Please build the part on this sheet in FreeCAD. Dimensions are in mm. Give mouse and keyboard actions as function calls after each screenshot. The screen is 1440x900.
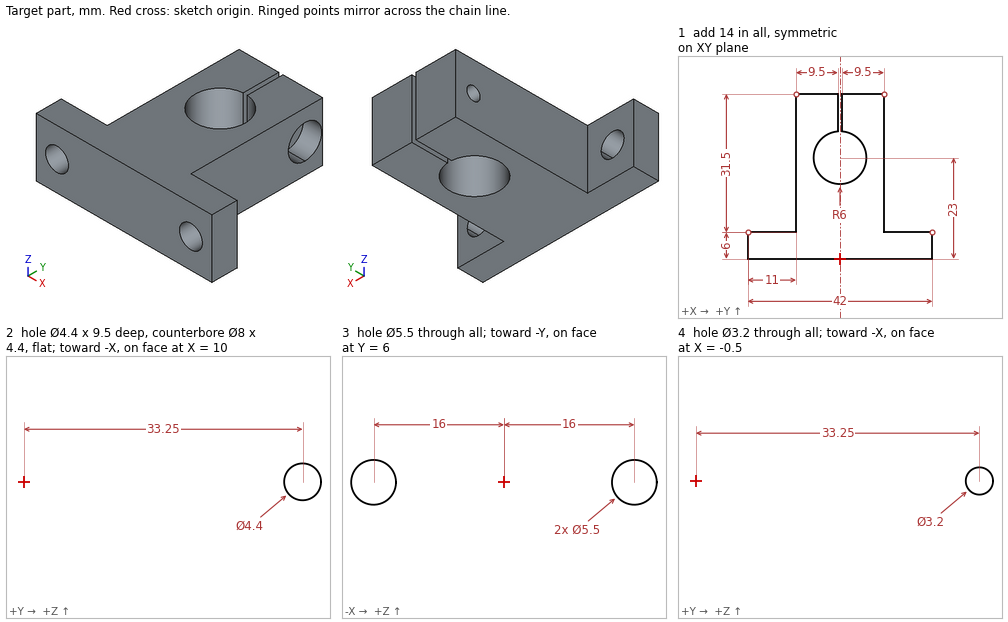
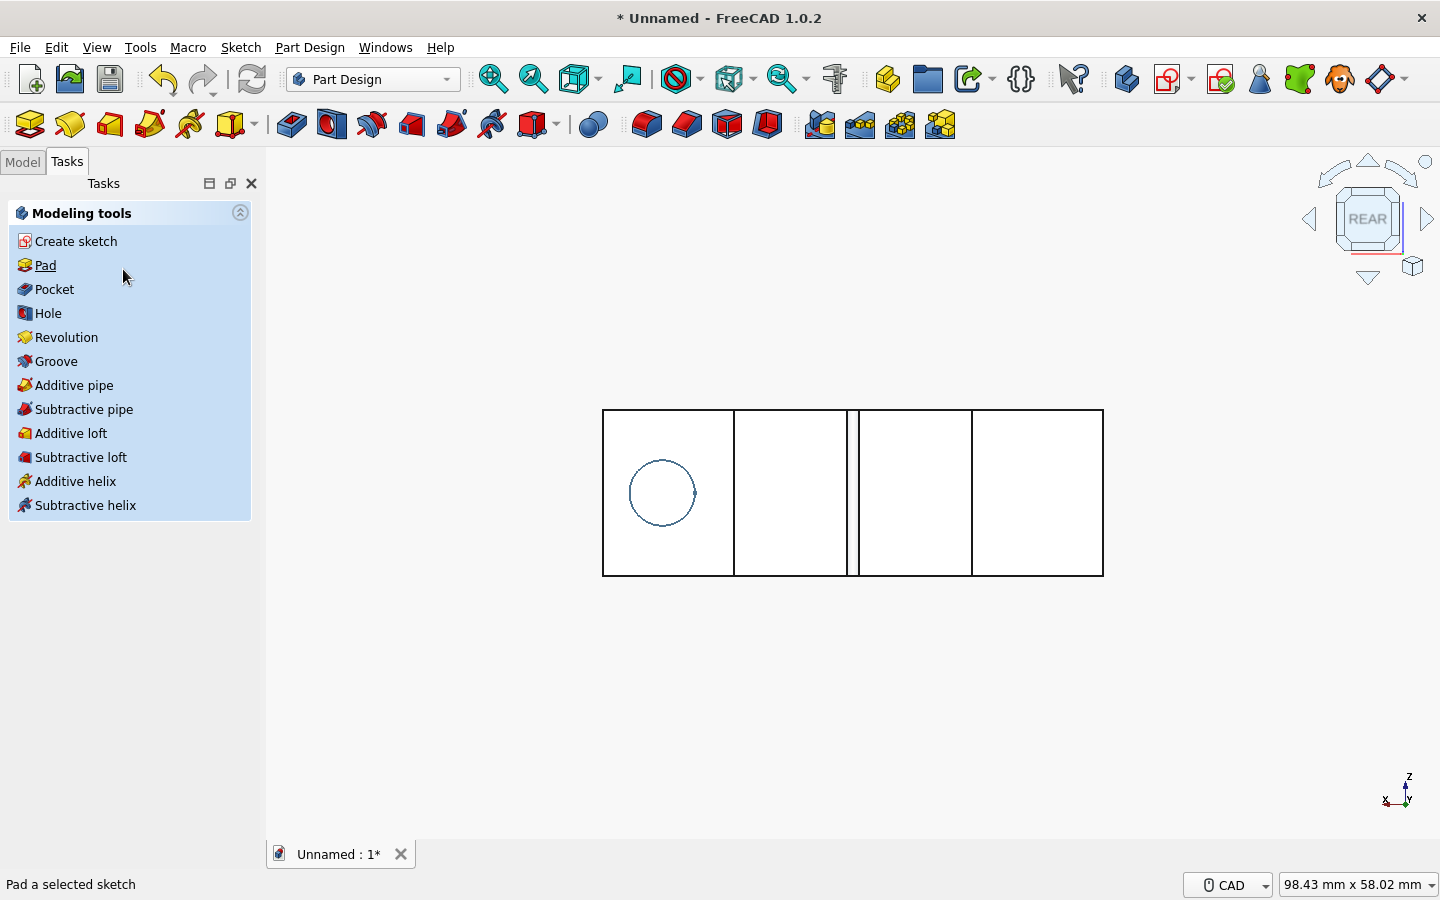
click(332, 124)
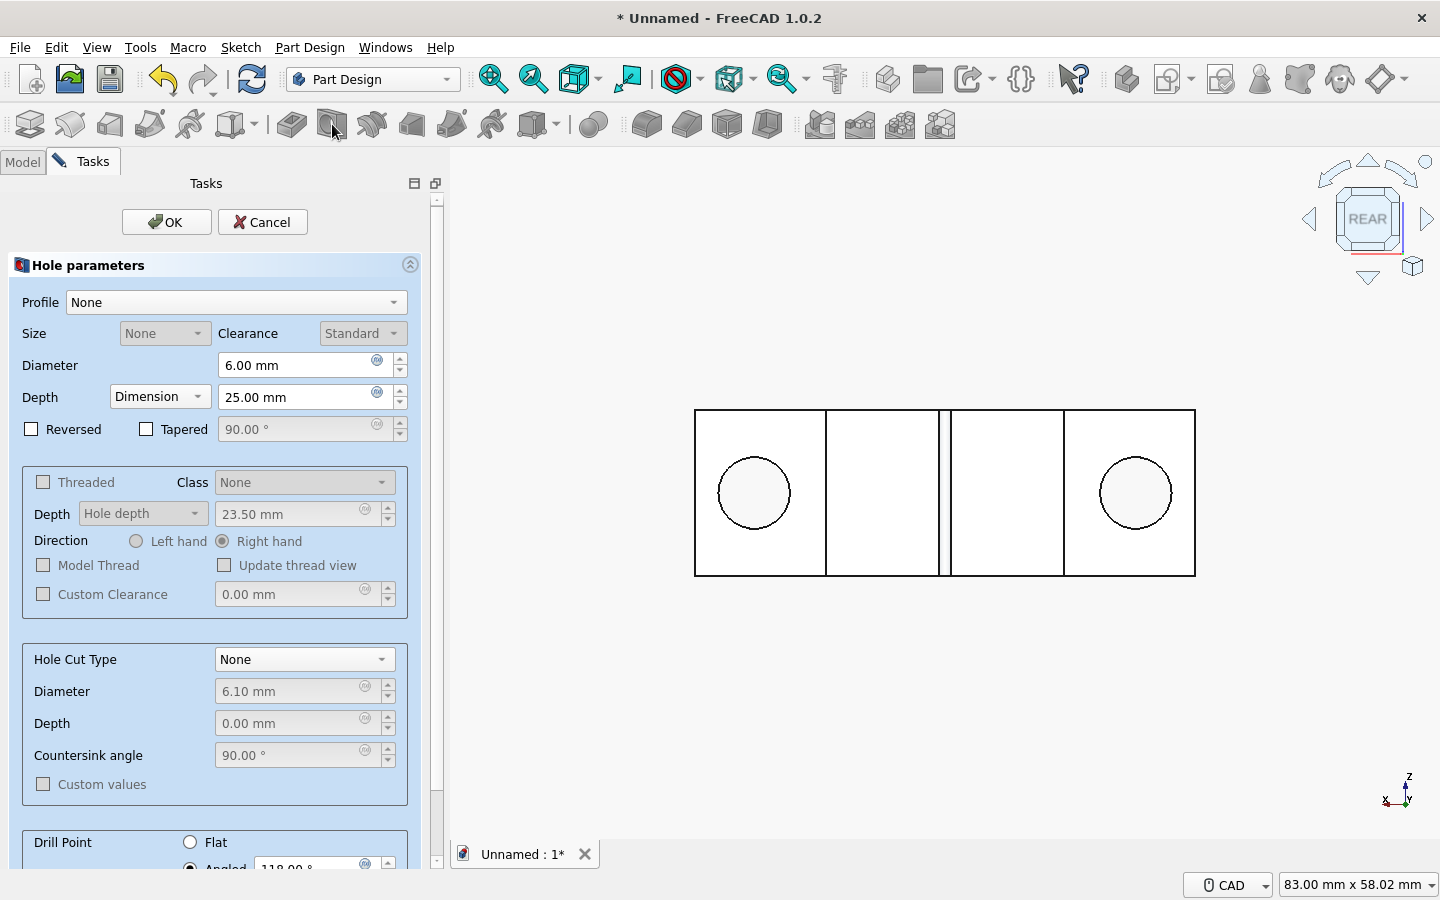
triple_click(305, 365)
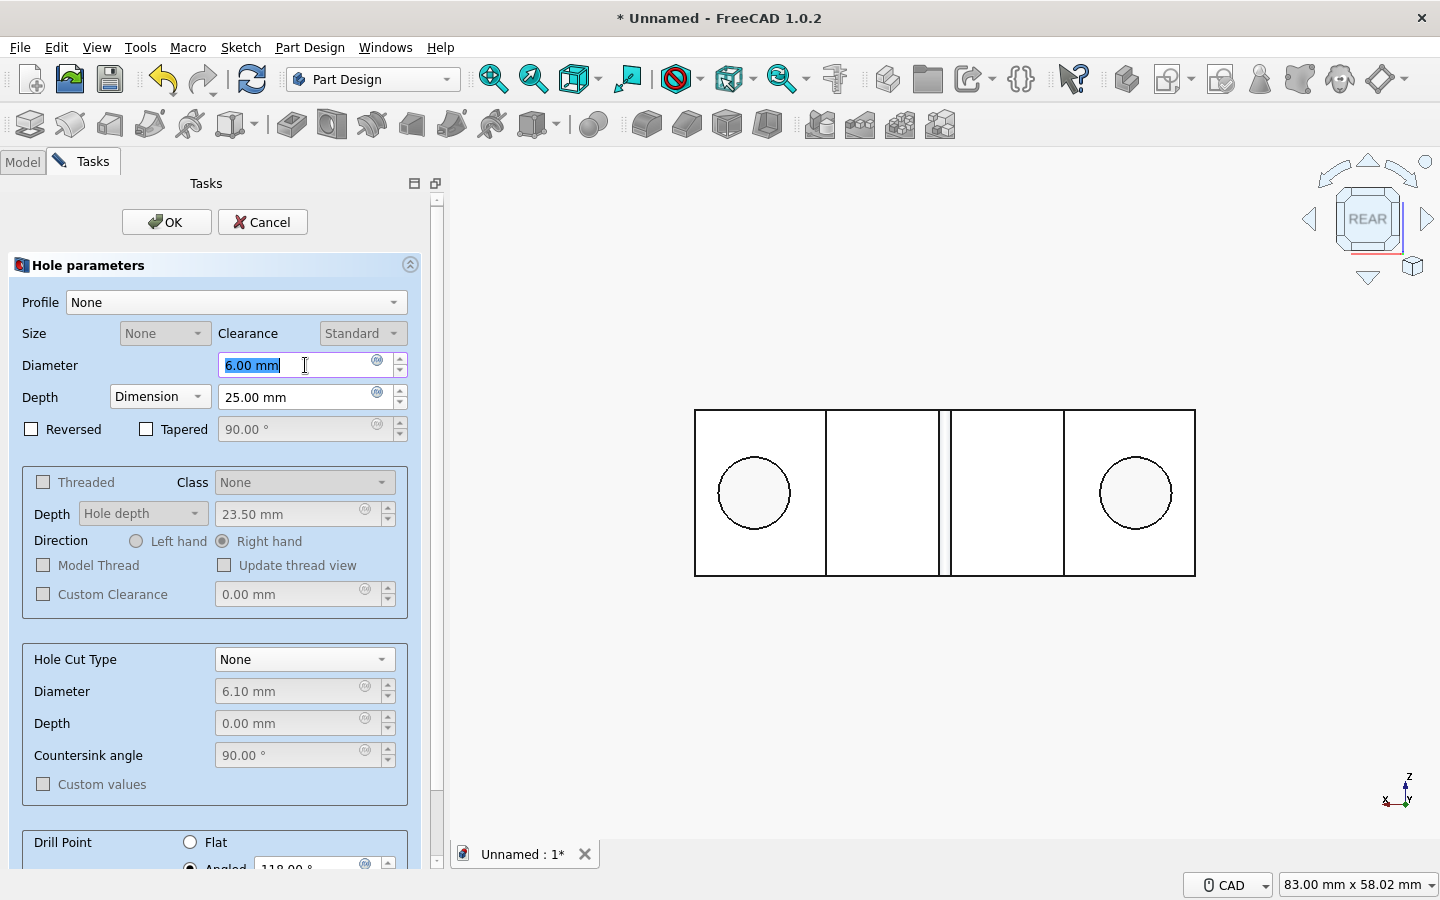
text(5.5)
key(Tab)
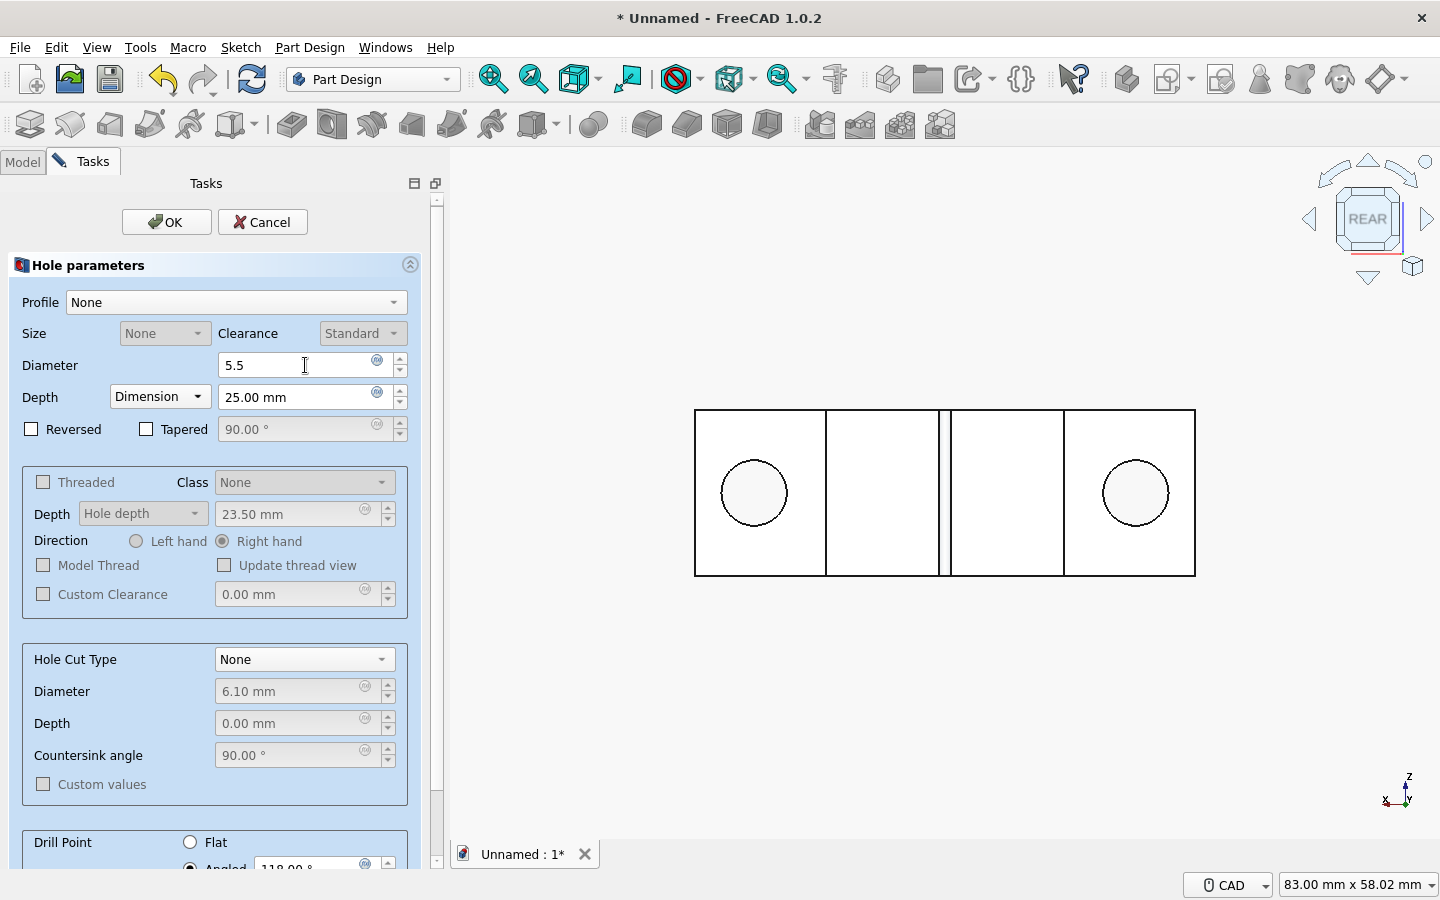
click(161, 396)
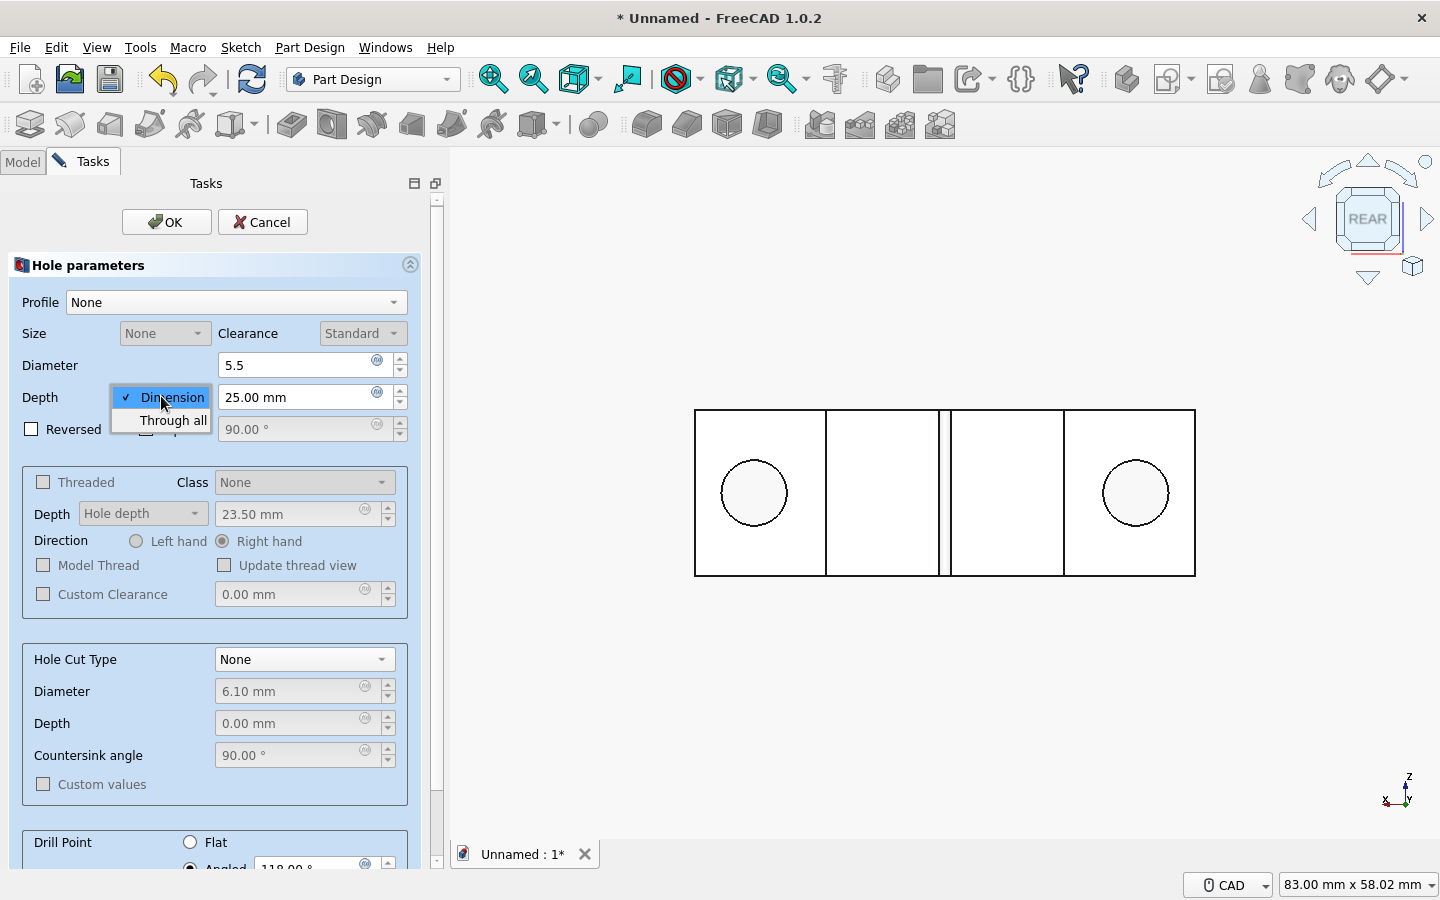
click(160, 420)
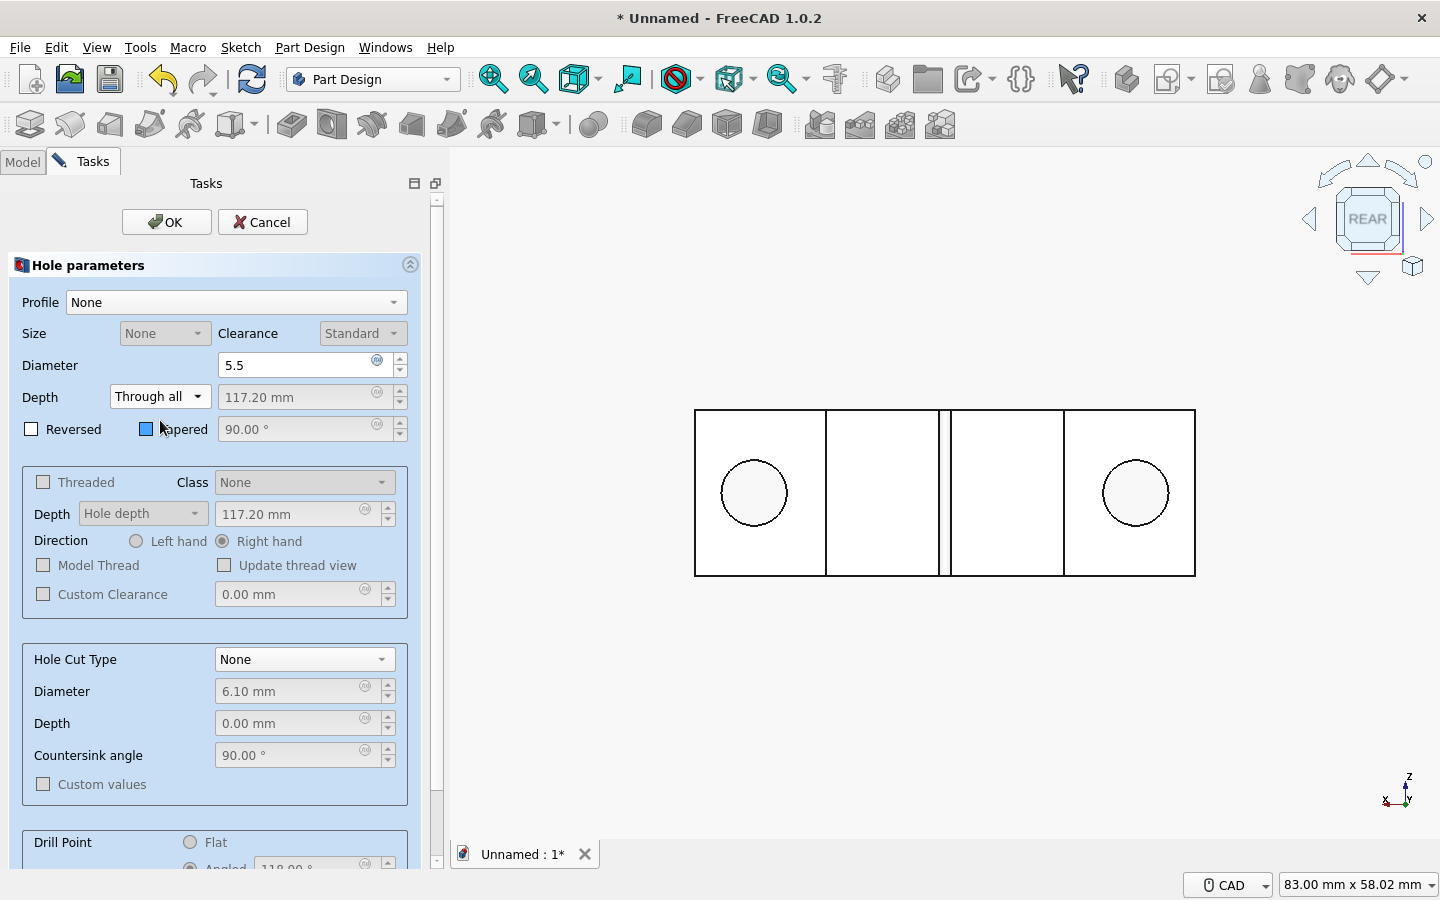
click(167, 222)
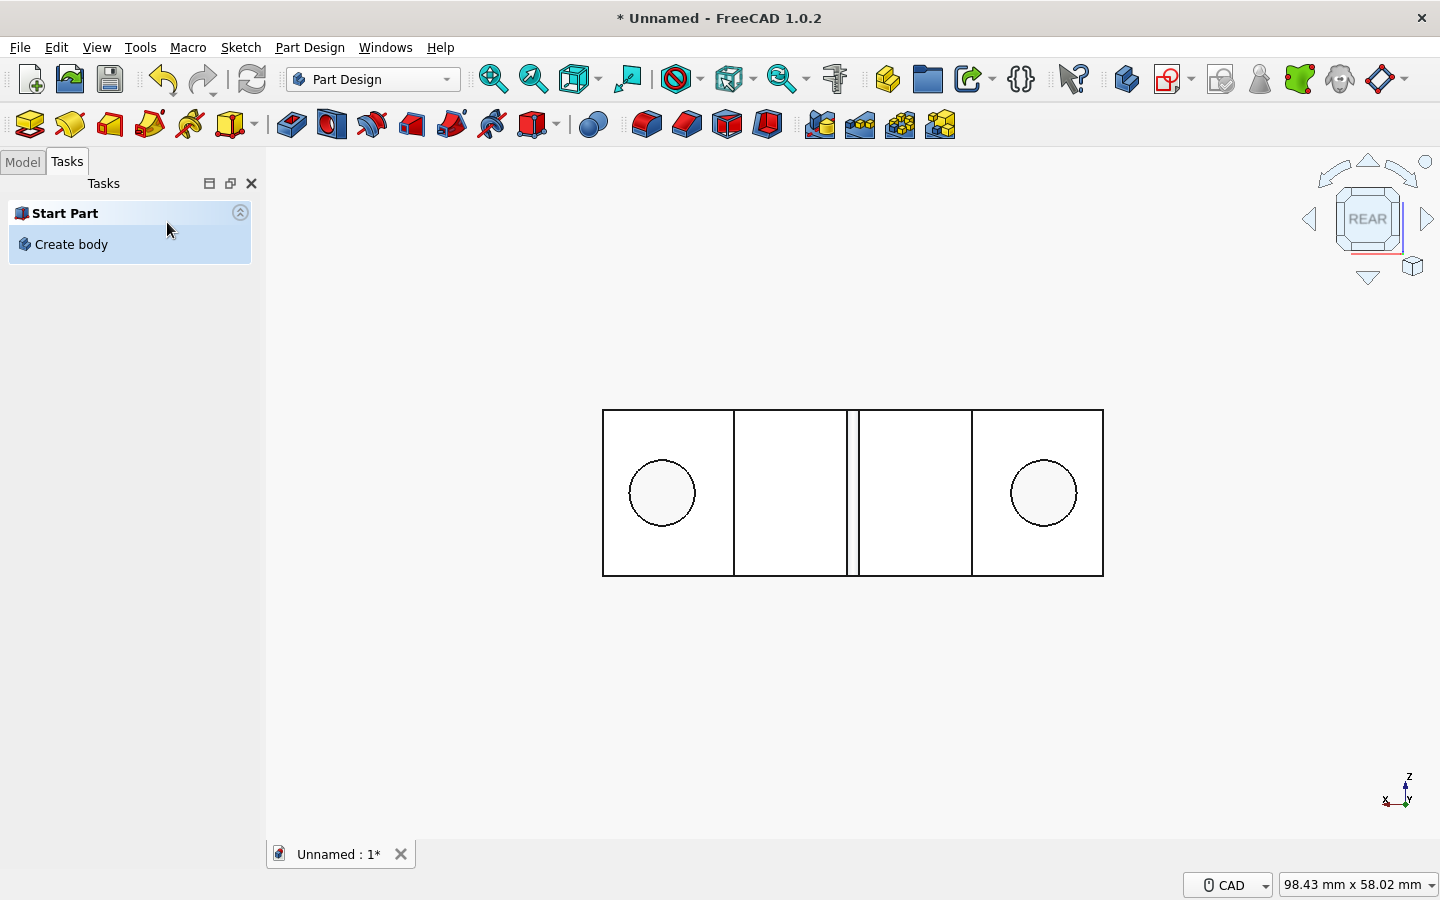
click(494, 80)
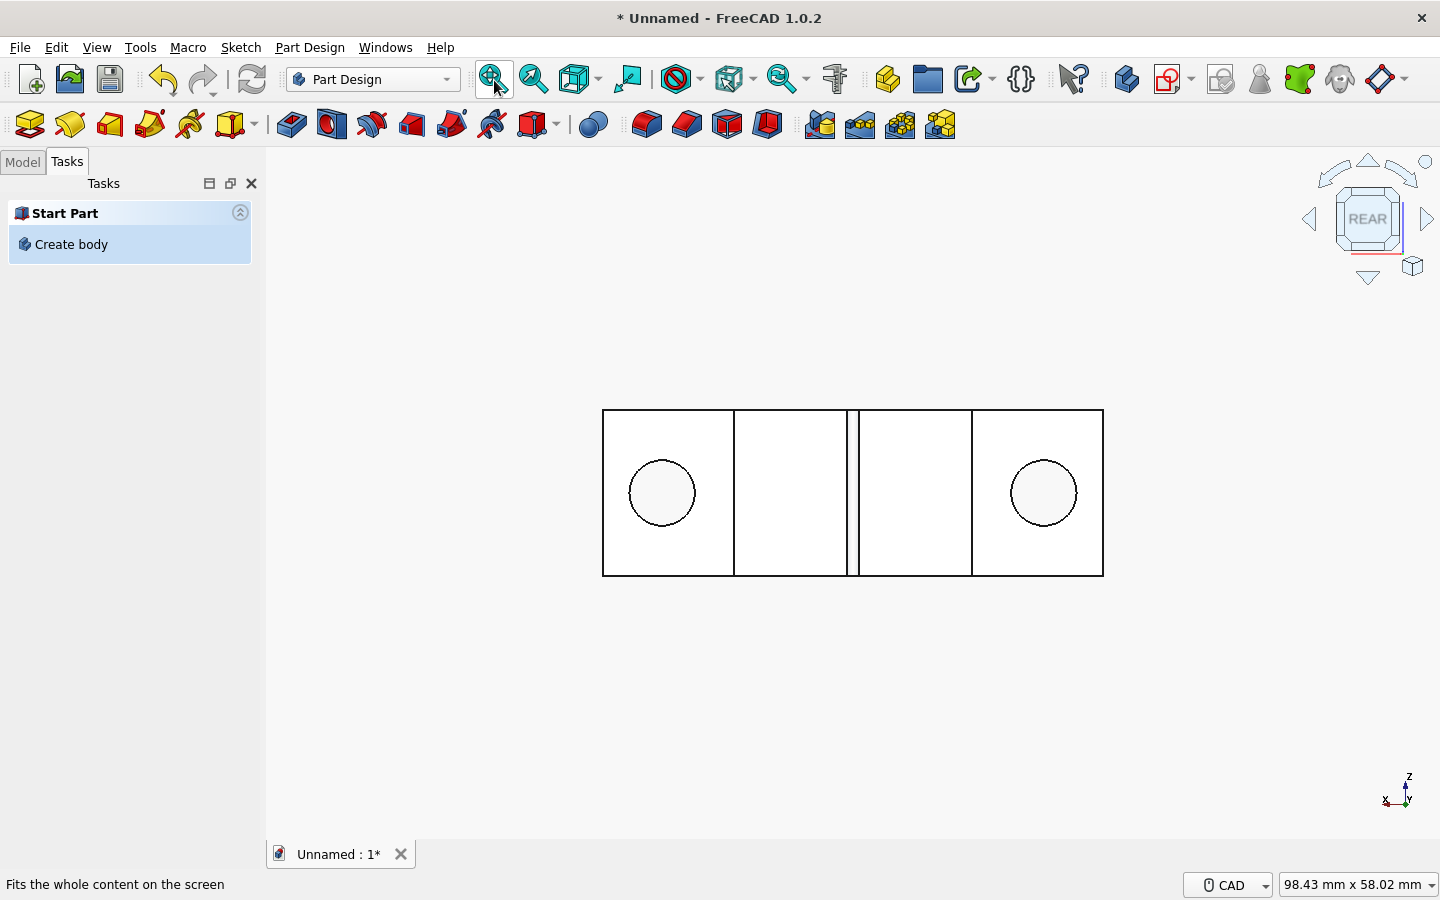
key(0)